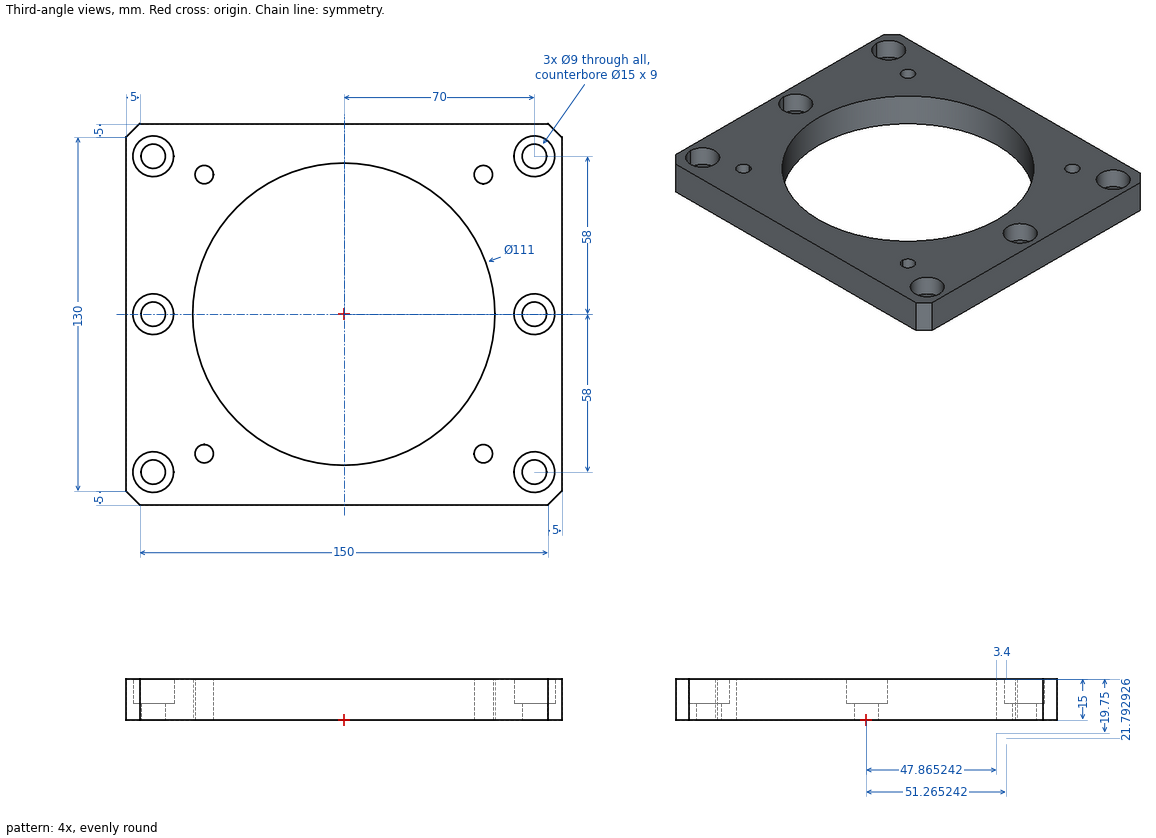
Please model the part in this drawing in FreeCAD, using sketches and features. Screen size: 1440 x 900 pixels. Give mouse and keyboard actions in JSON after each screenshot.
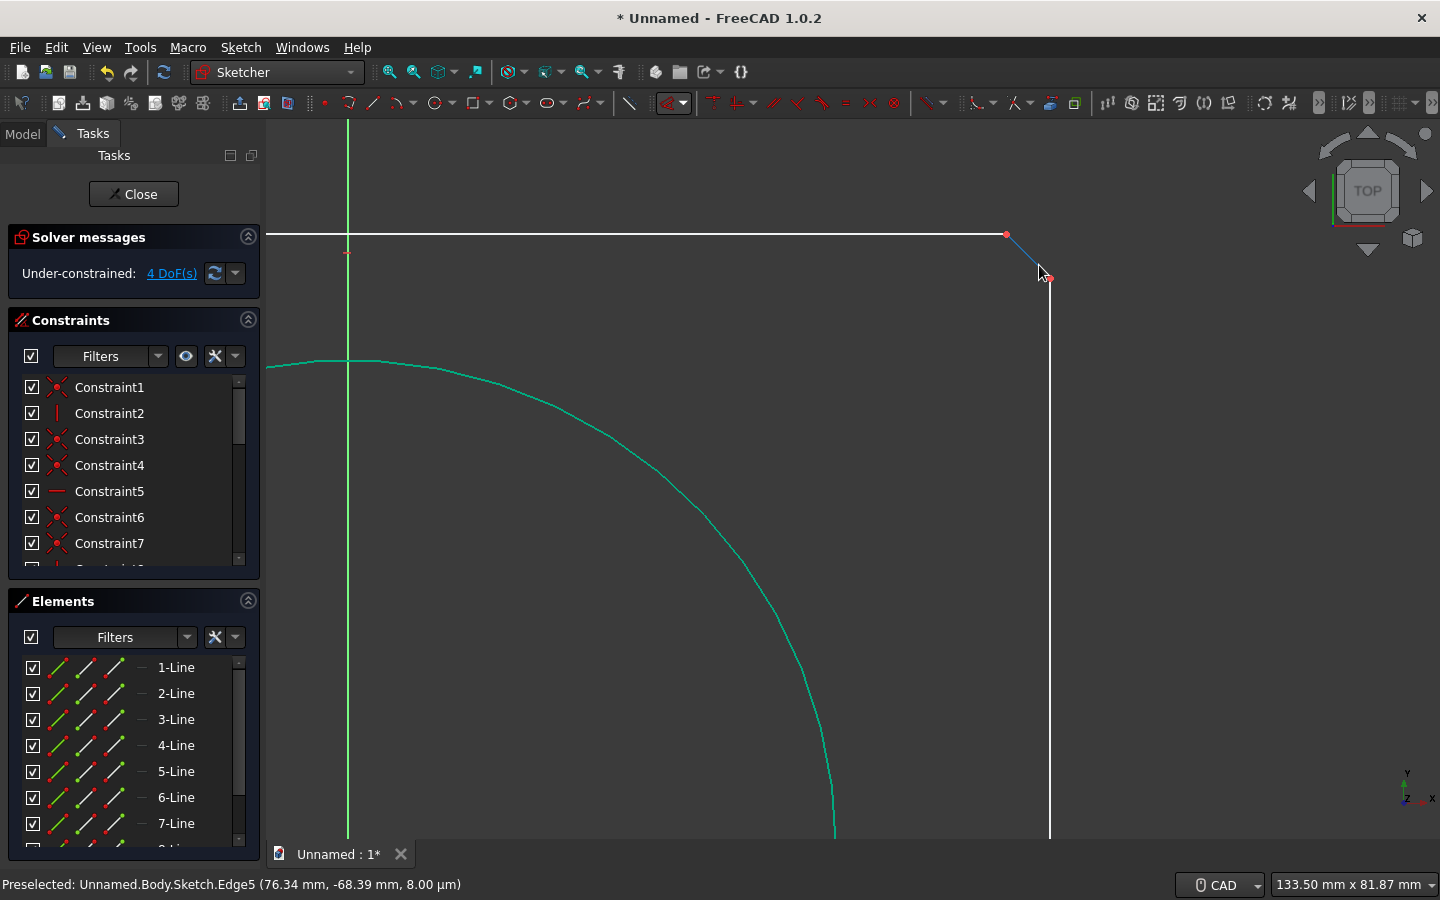
{"action": "left_click", "coordinate": [1037, 265]}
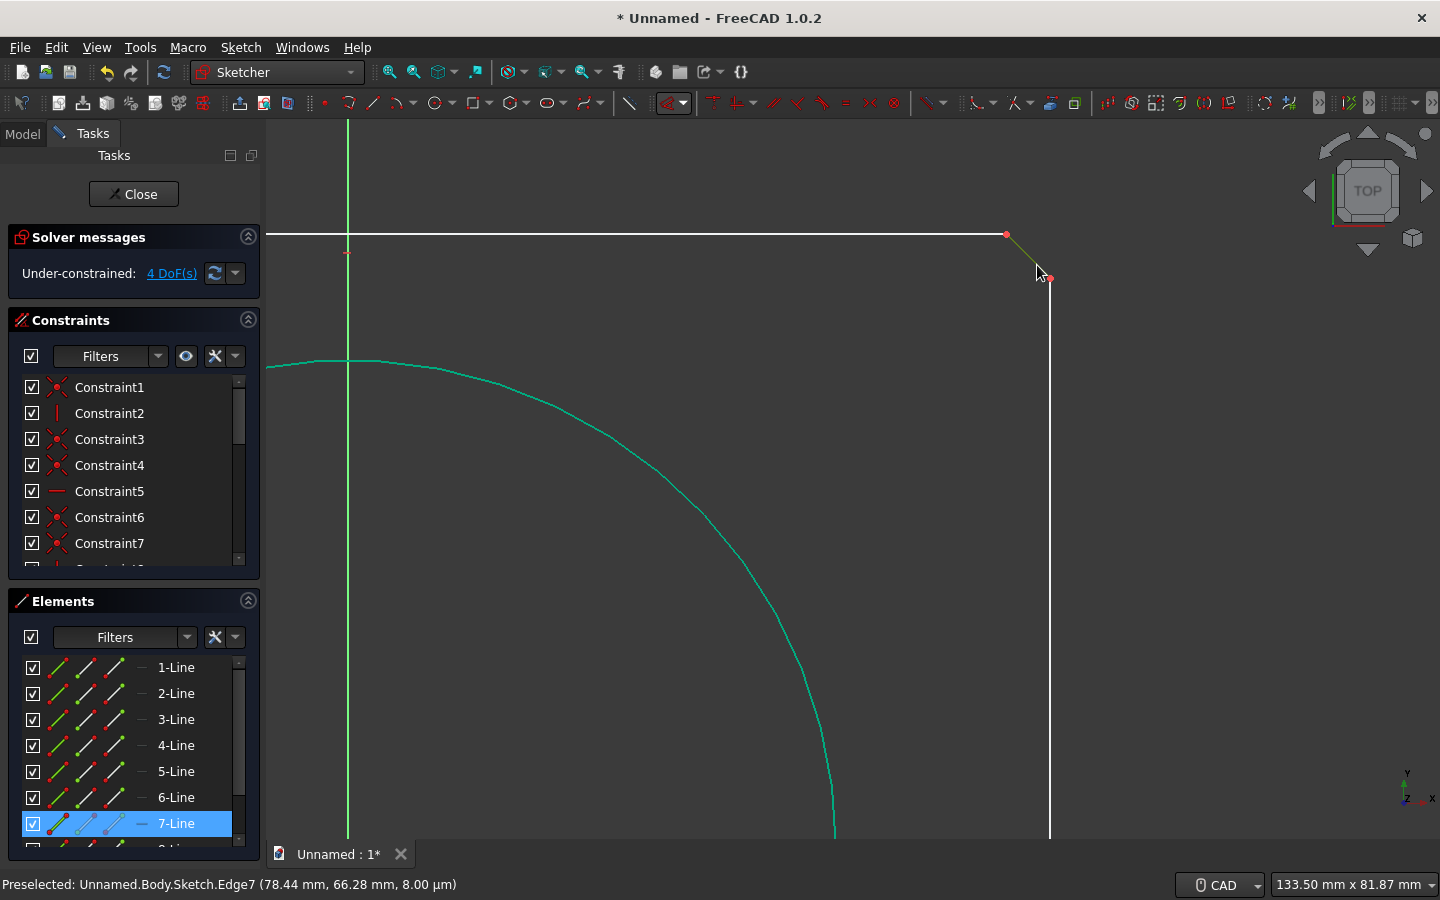
{"action": "key", "text": "l"}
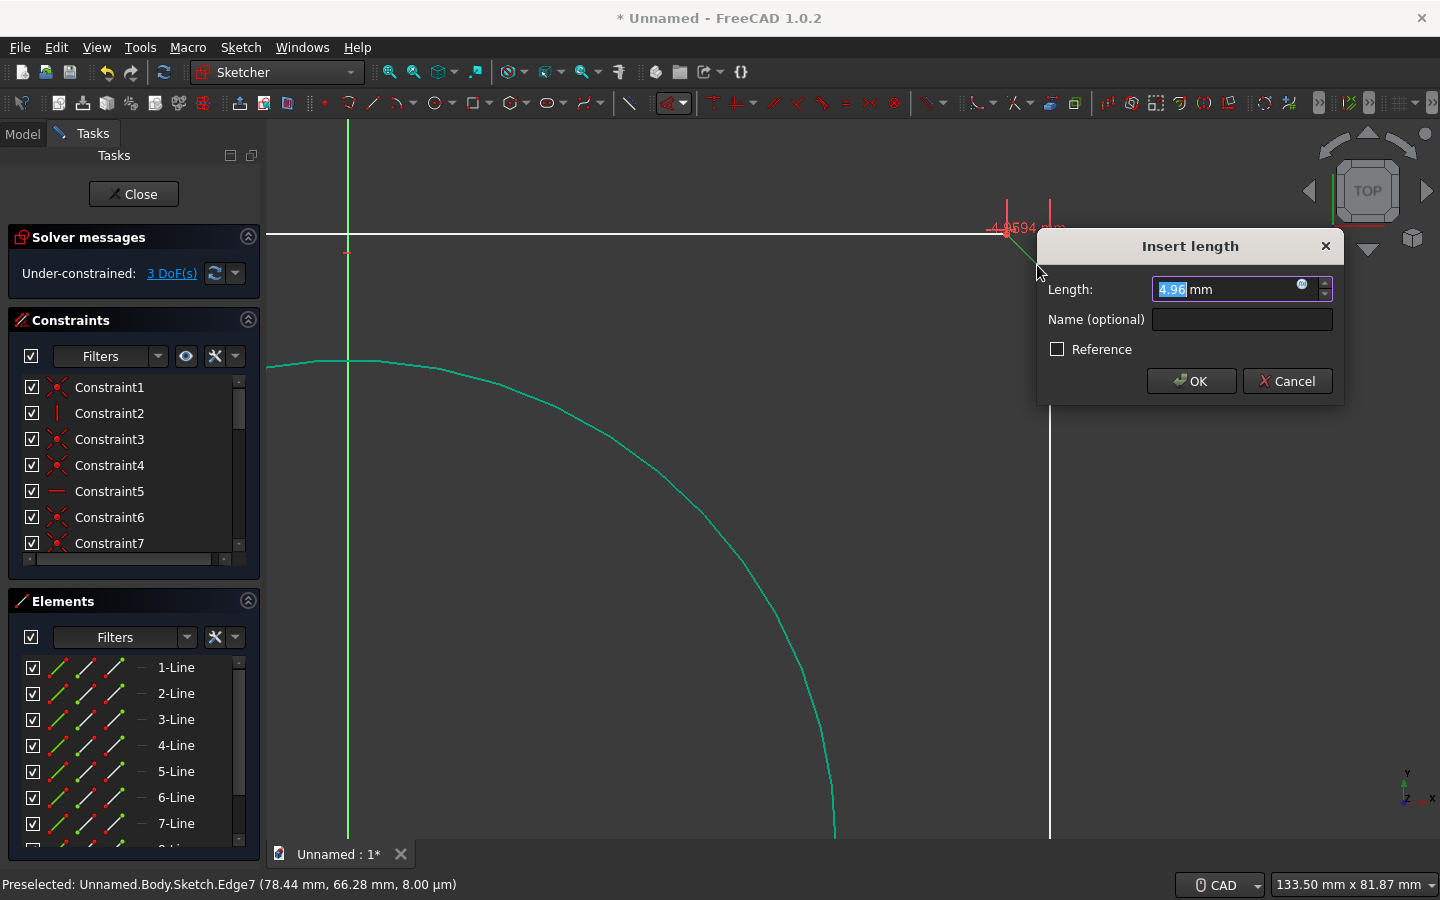
{"action": "type", "text": "5"}
{"action": "key", "text": "Return"}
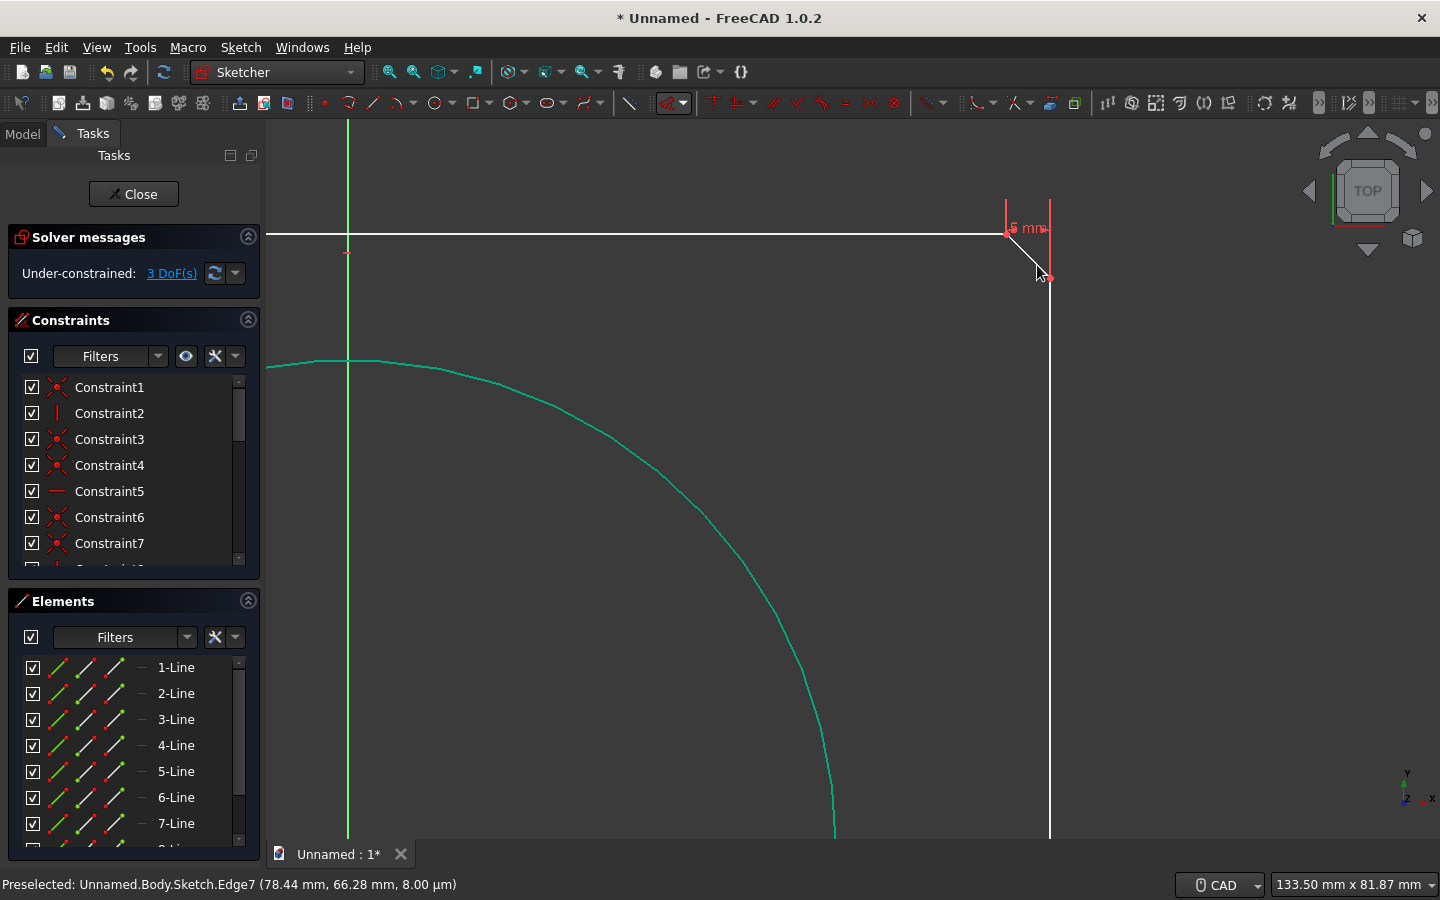
{"action": "left_click", "coordinate": [1037, 265]}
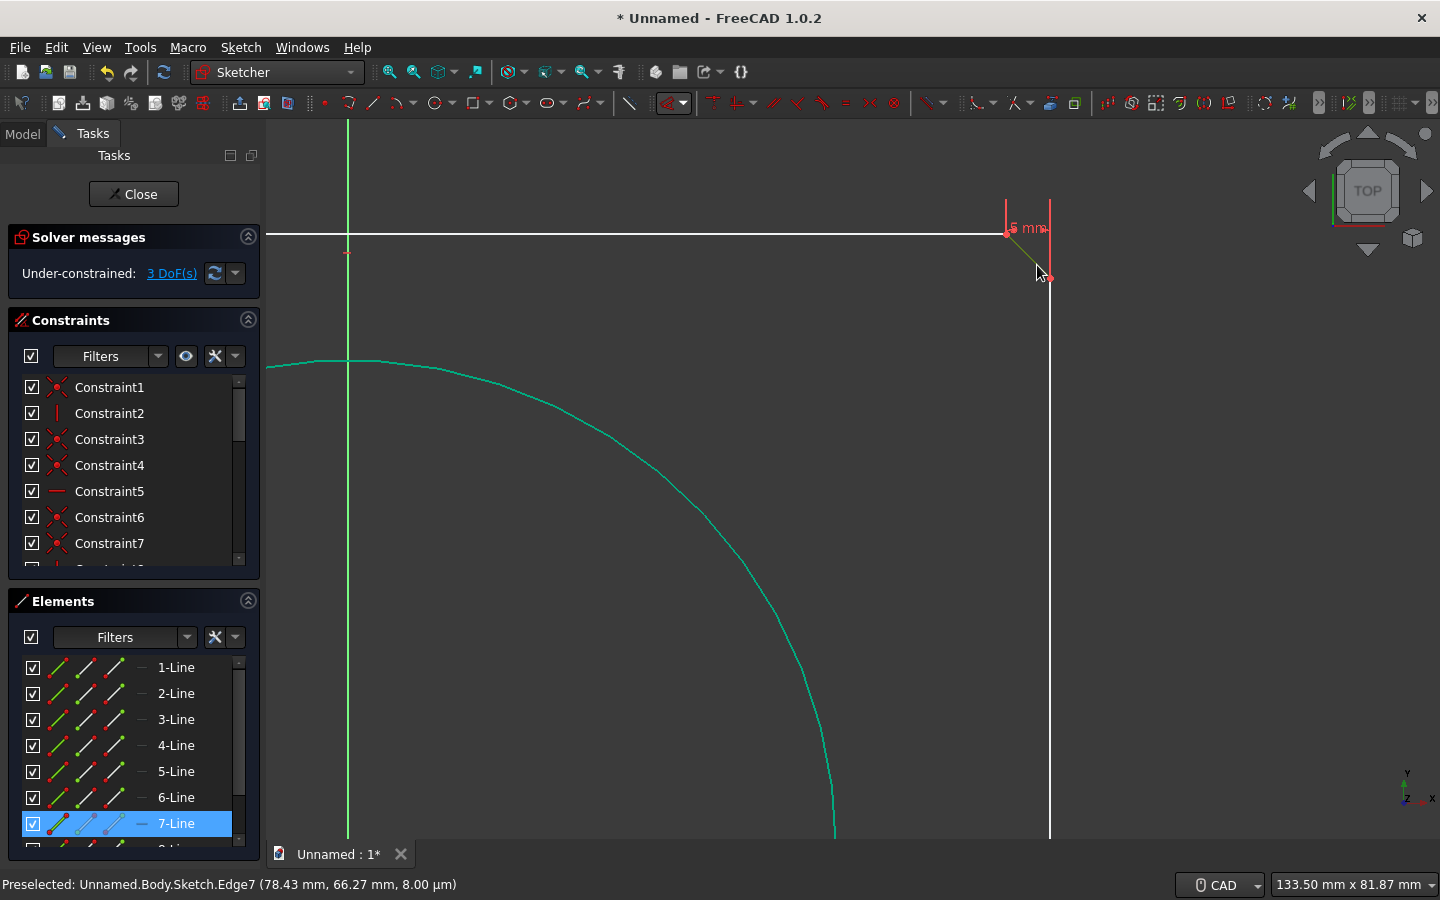
{"action": "key", "text": "i"}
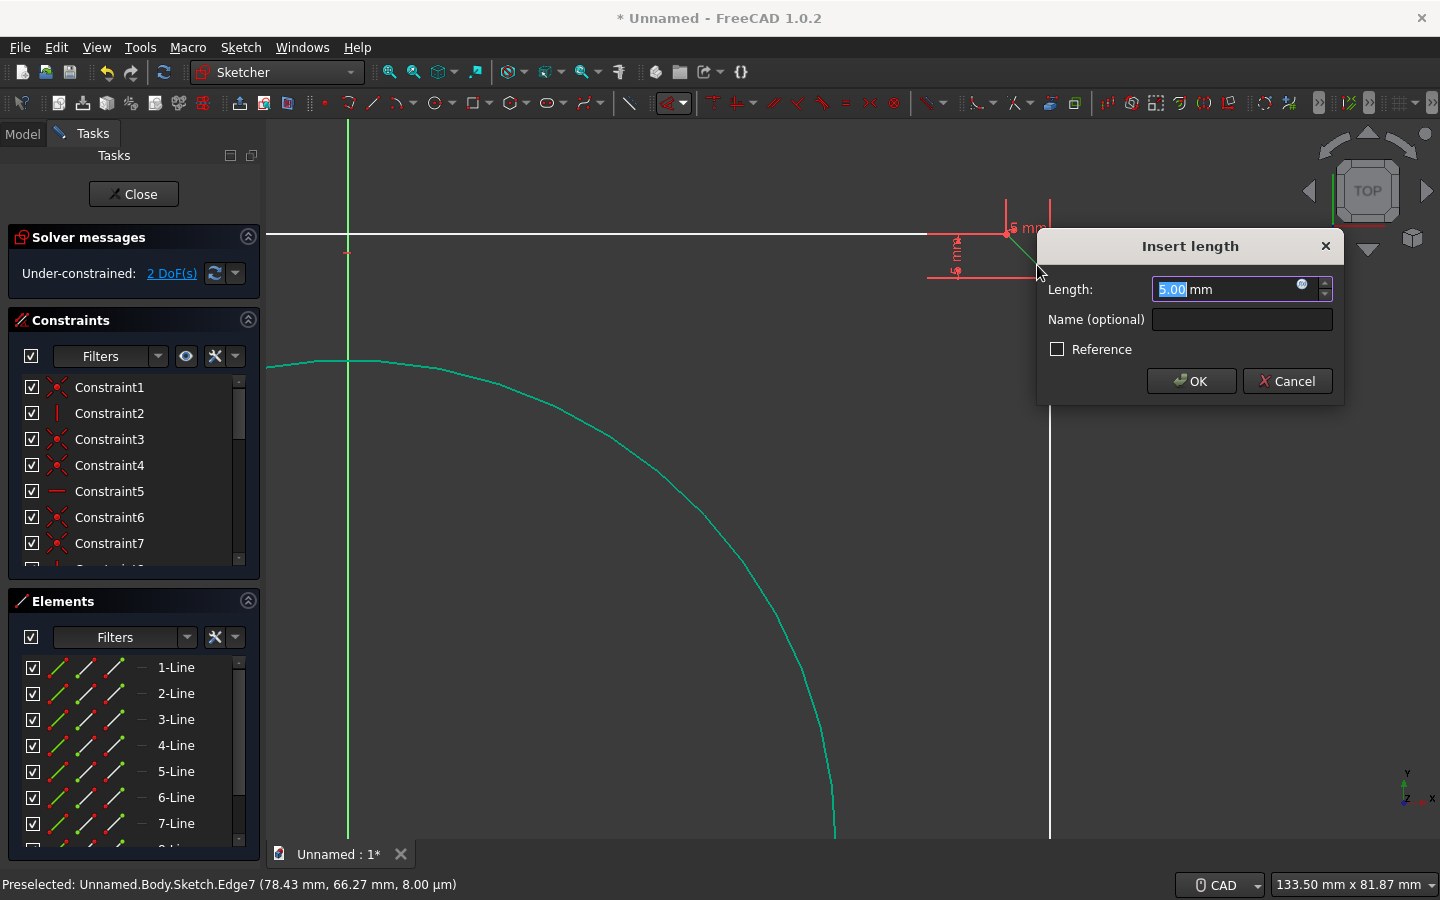
{"action": "type", "text": "5"}
{"action": "key", "text": "Return"}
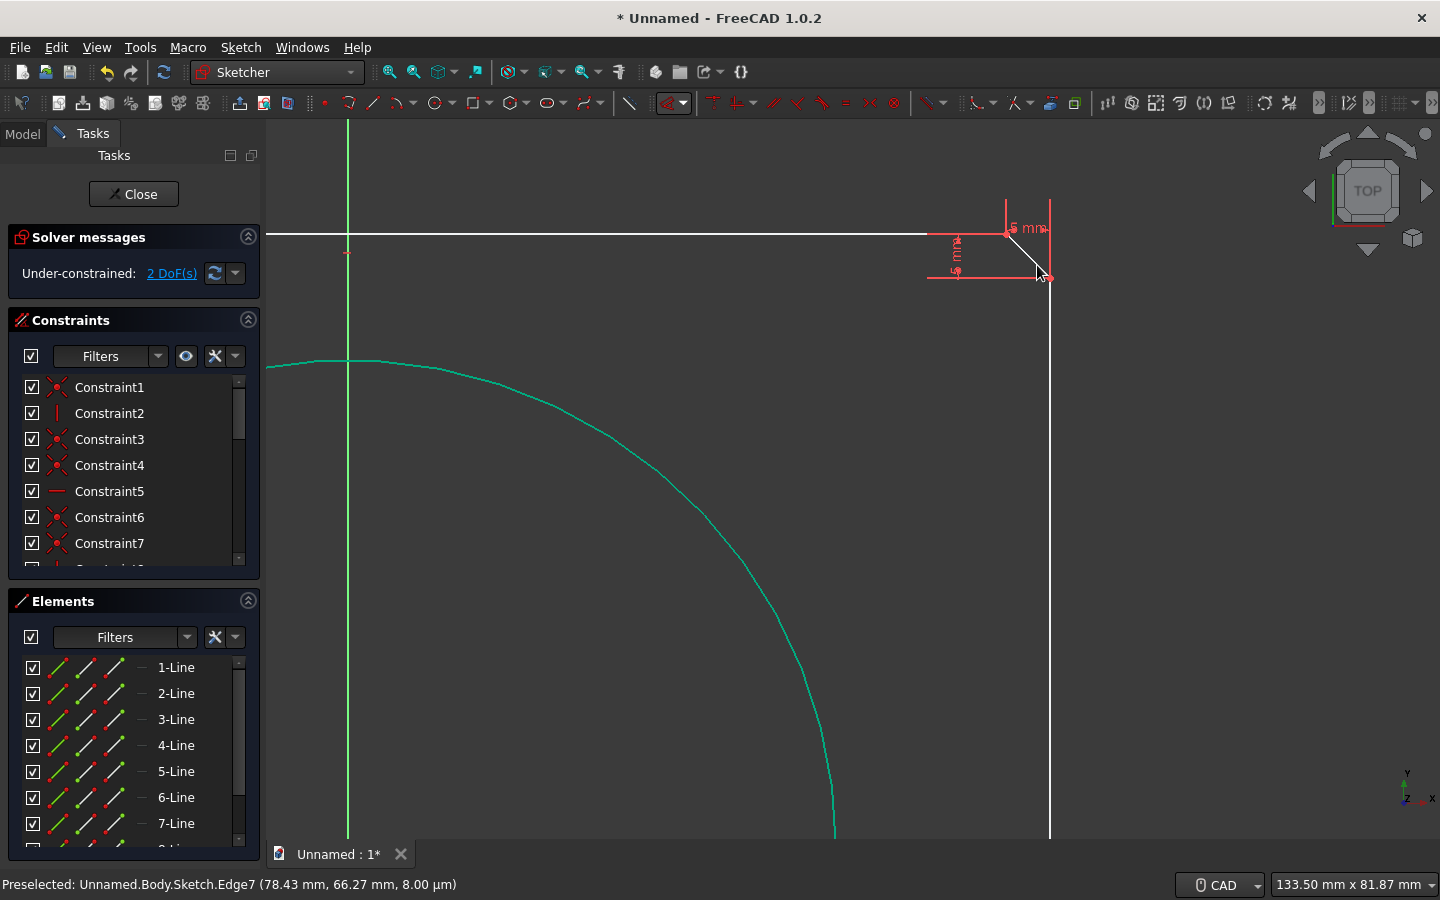
{"action": "scroll", "coordinate": [1039, 264], "scroll_direction": "down", "scroll_amount": 5}